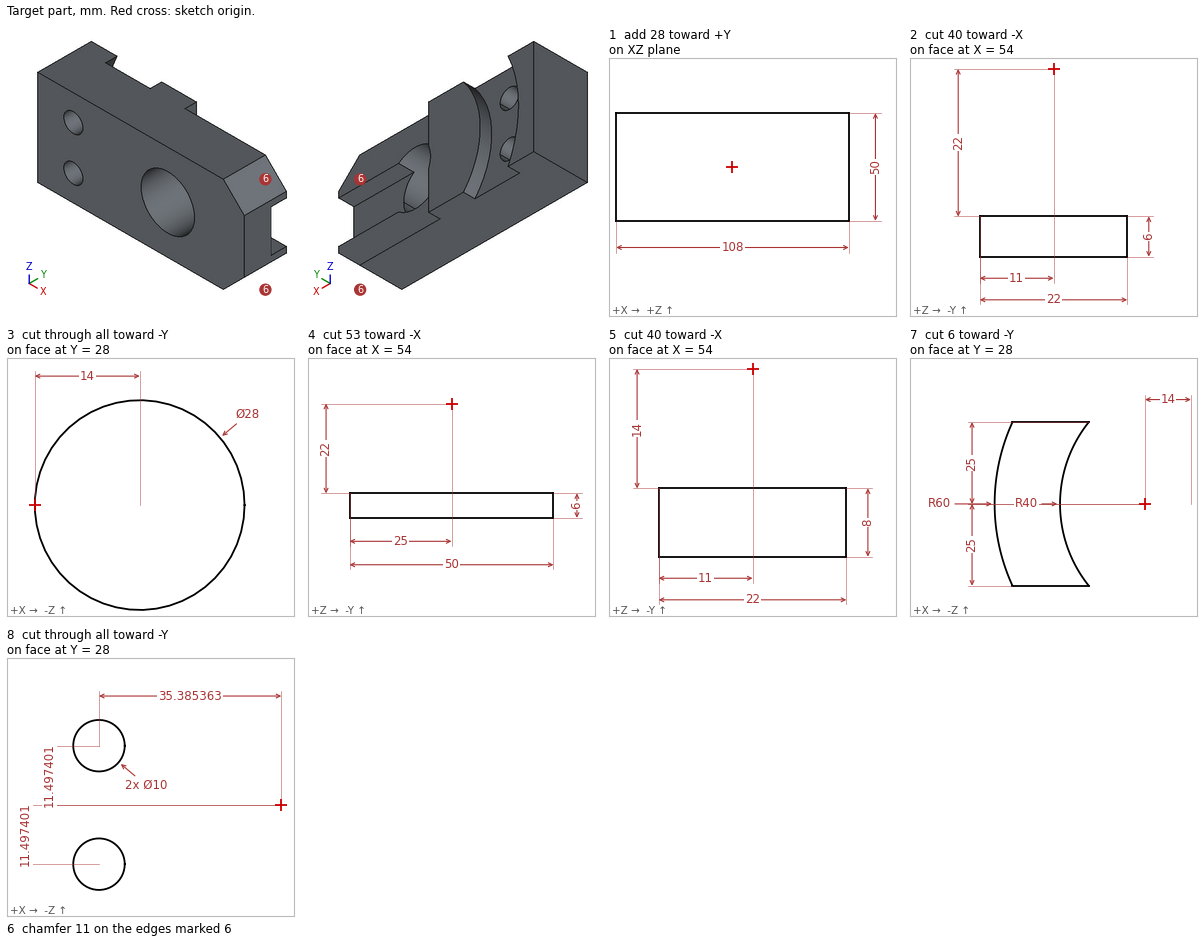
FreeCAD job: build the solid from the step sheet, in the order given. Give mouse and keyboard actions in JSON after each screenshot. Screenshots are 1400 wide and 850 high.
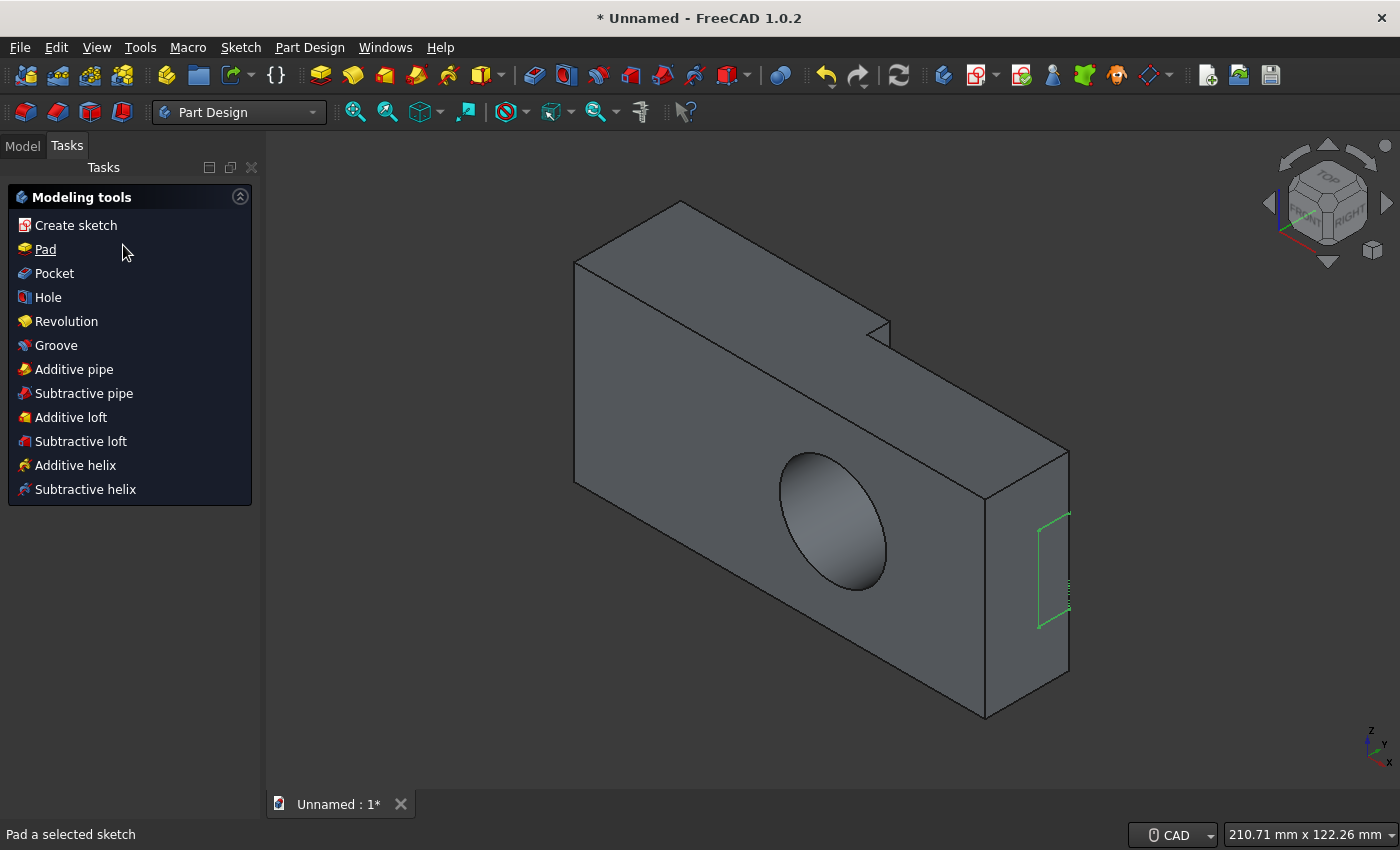
{"action": "left_click", "coordinate": [536, 76]}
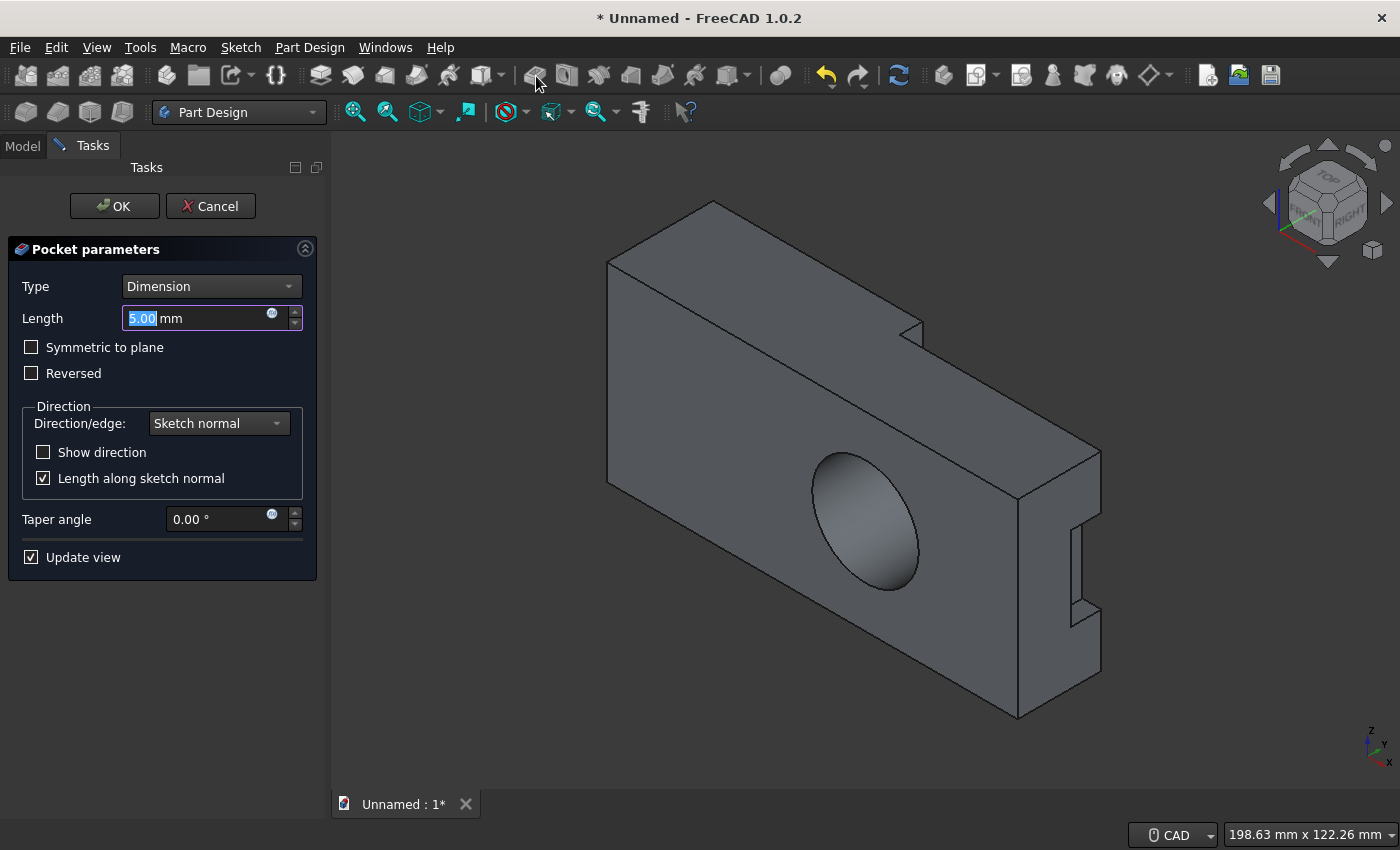
{"action": "type", "text": "40"}
{"action": "key", "text": "Tab"}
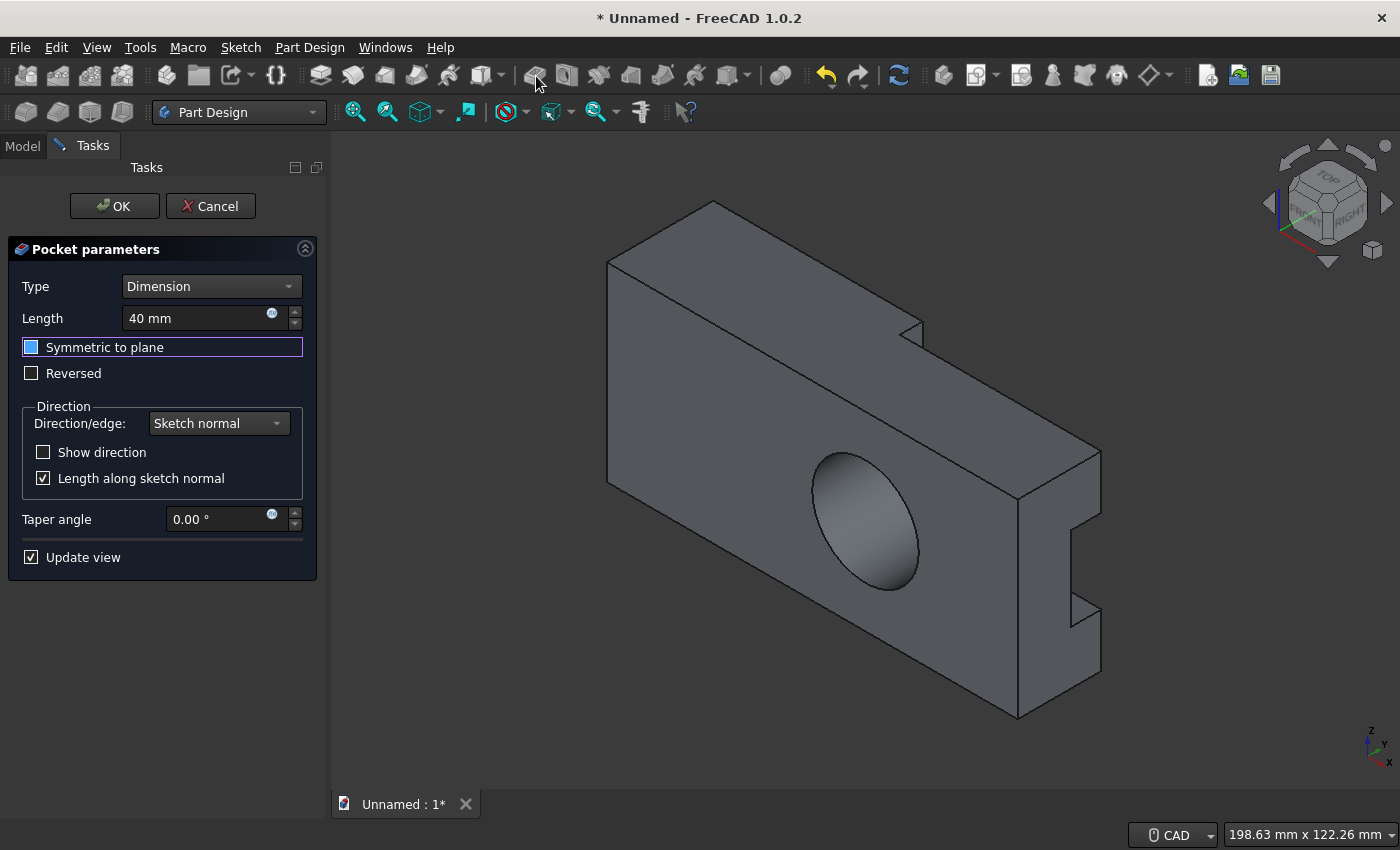
{"action": "left_click", "coordinate": [115, 206]}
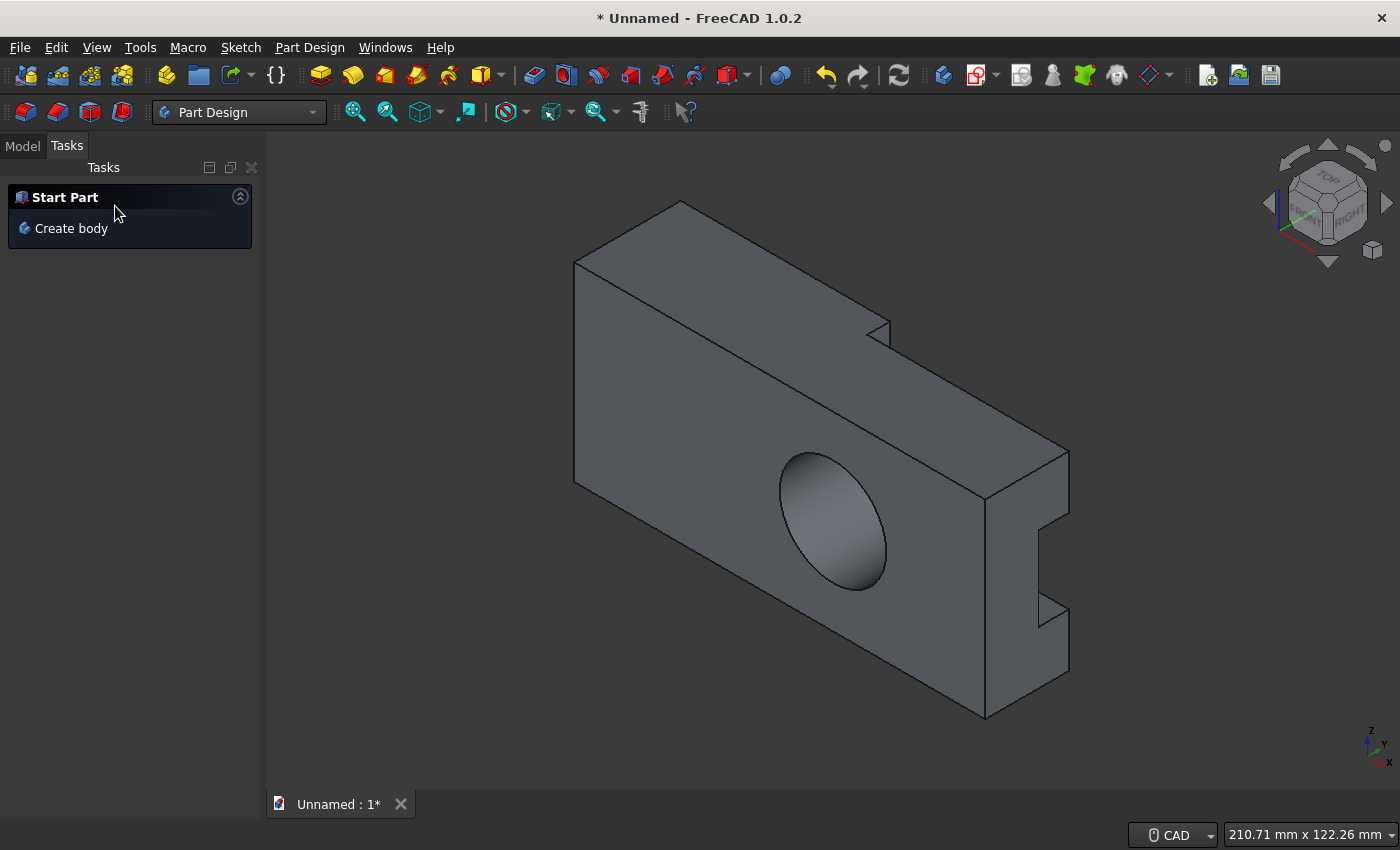
{"action": "left_click", "coordinate": [1027, 474]}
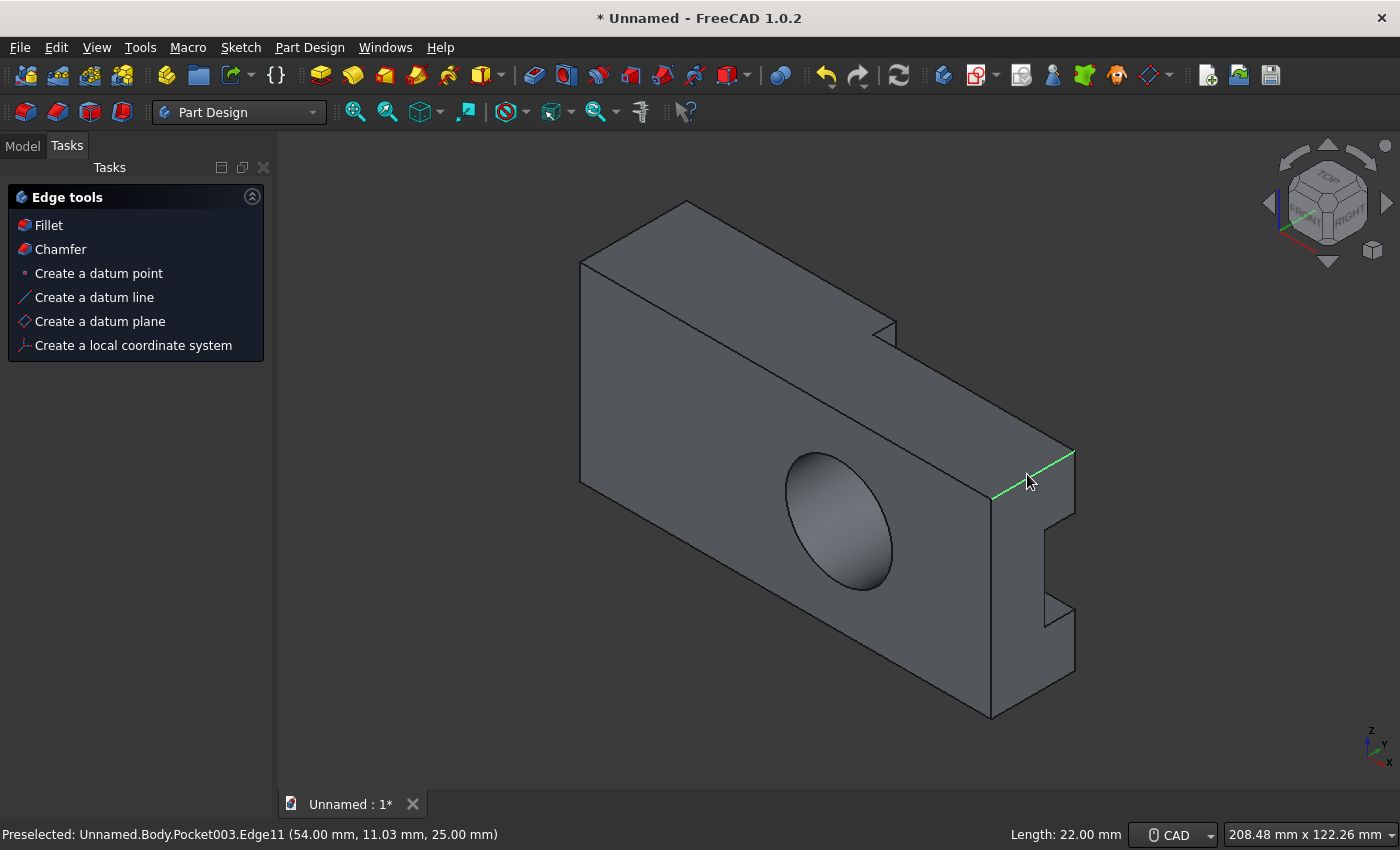
{"action": "key", "text": "2"}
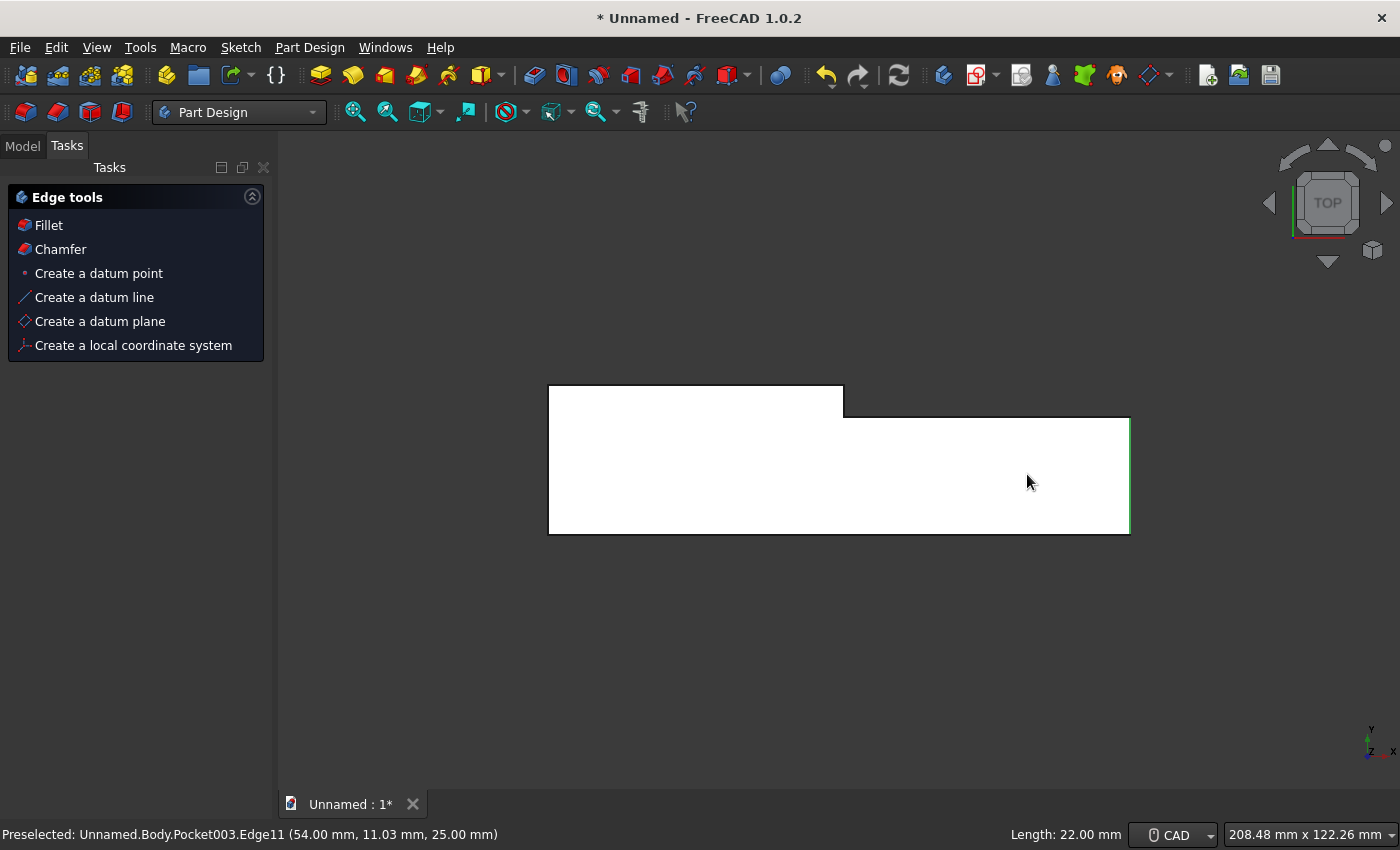
{"action": "key", "text": "0"}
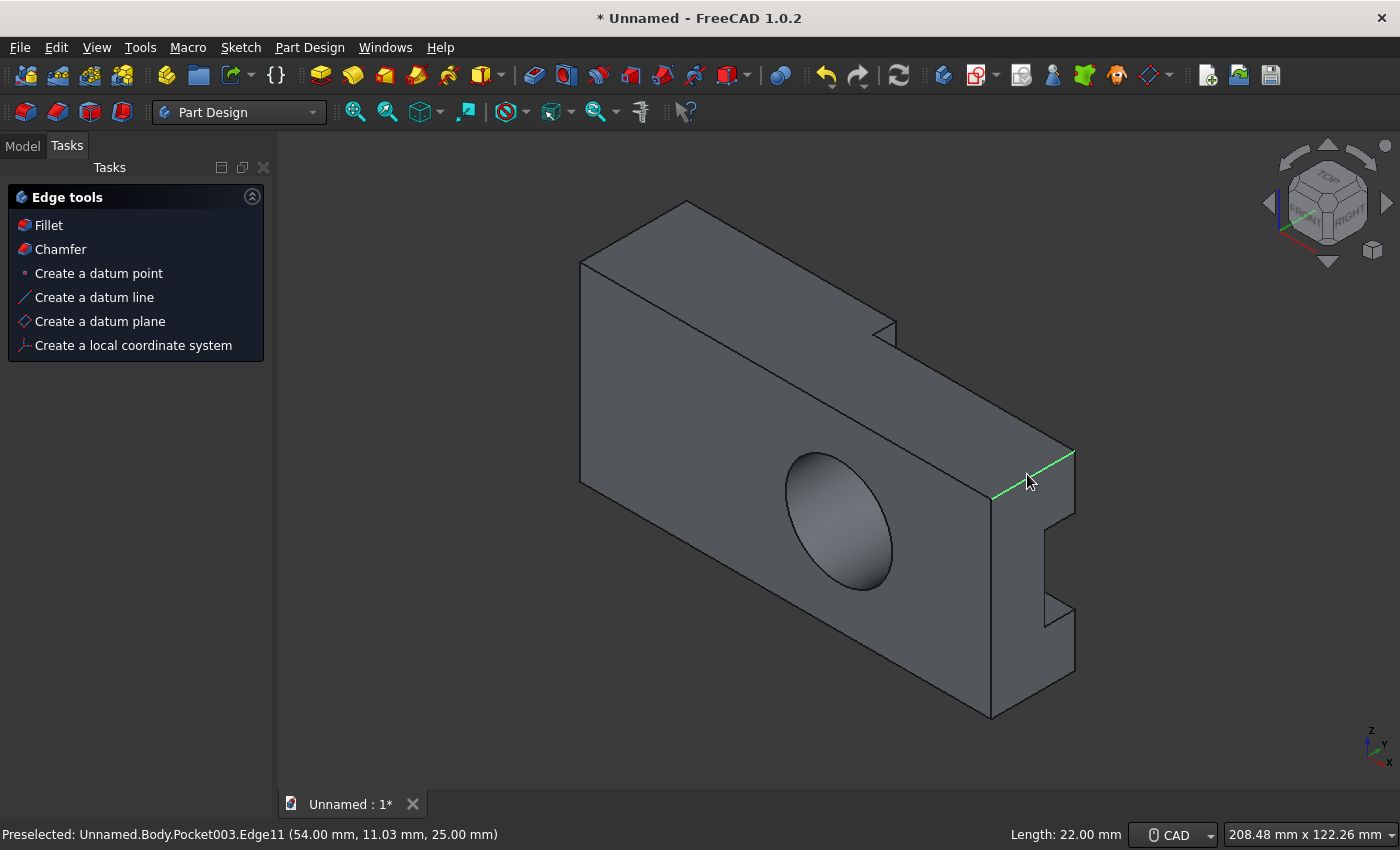
{"action": "key", "text": "1"}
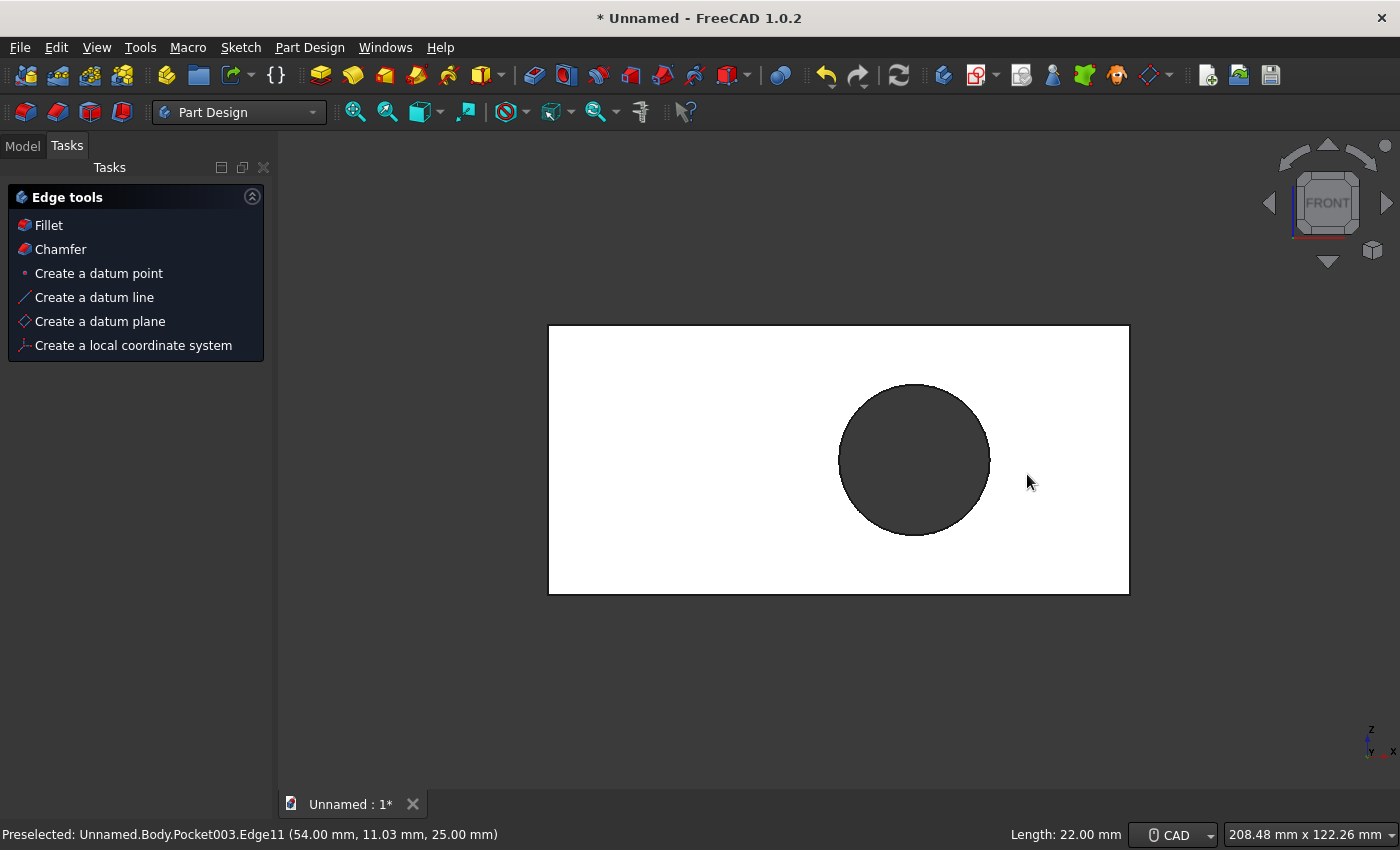
{"action": "key", "text": "3"}